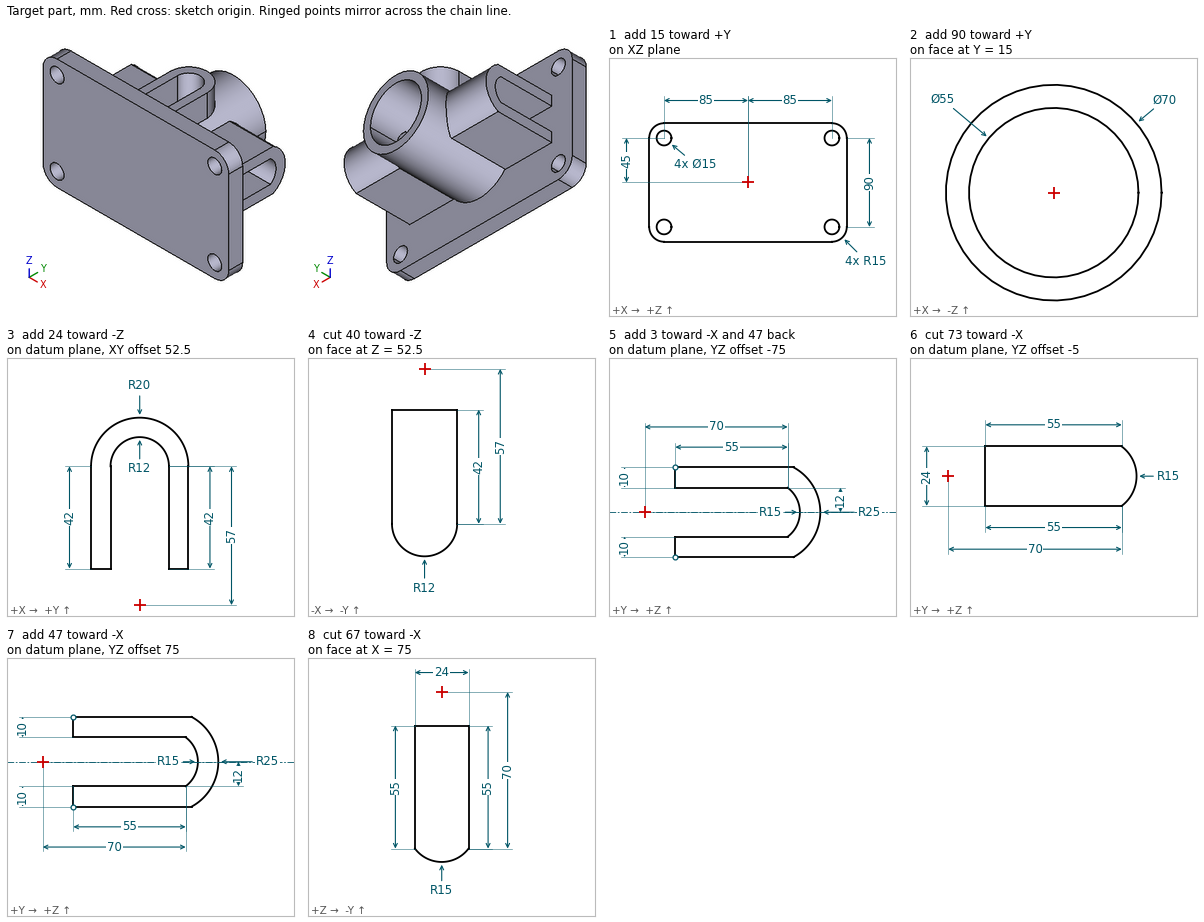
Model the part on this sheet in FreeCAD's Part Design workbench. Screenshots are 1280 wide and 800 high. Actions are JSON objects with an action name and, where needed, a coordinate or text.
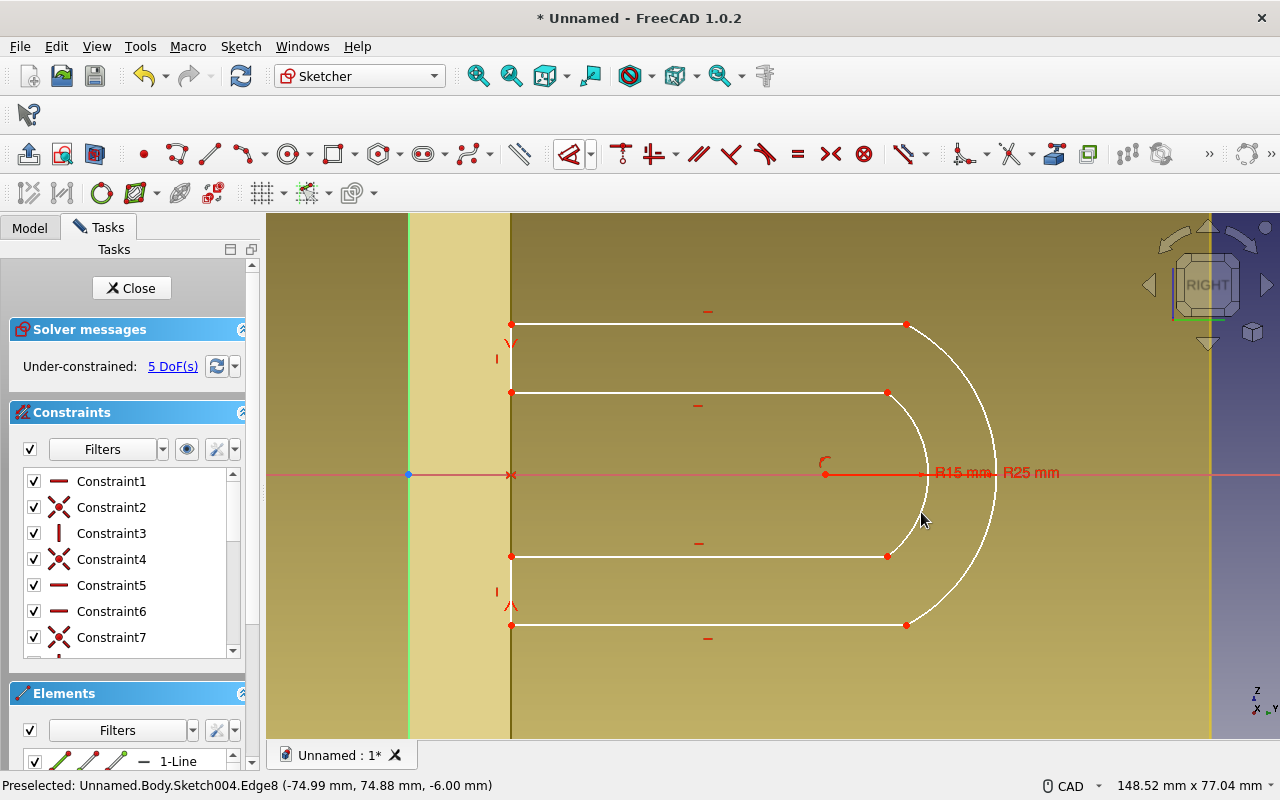
{"action": "left_click", "coordinate": [774, 393]}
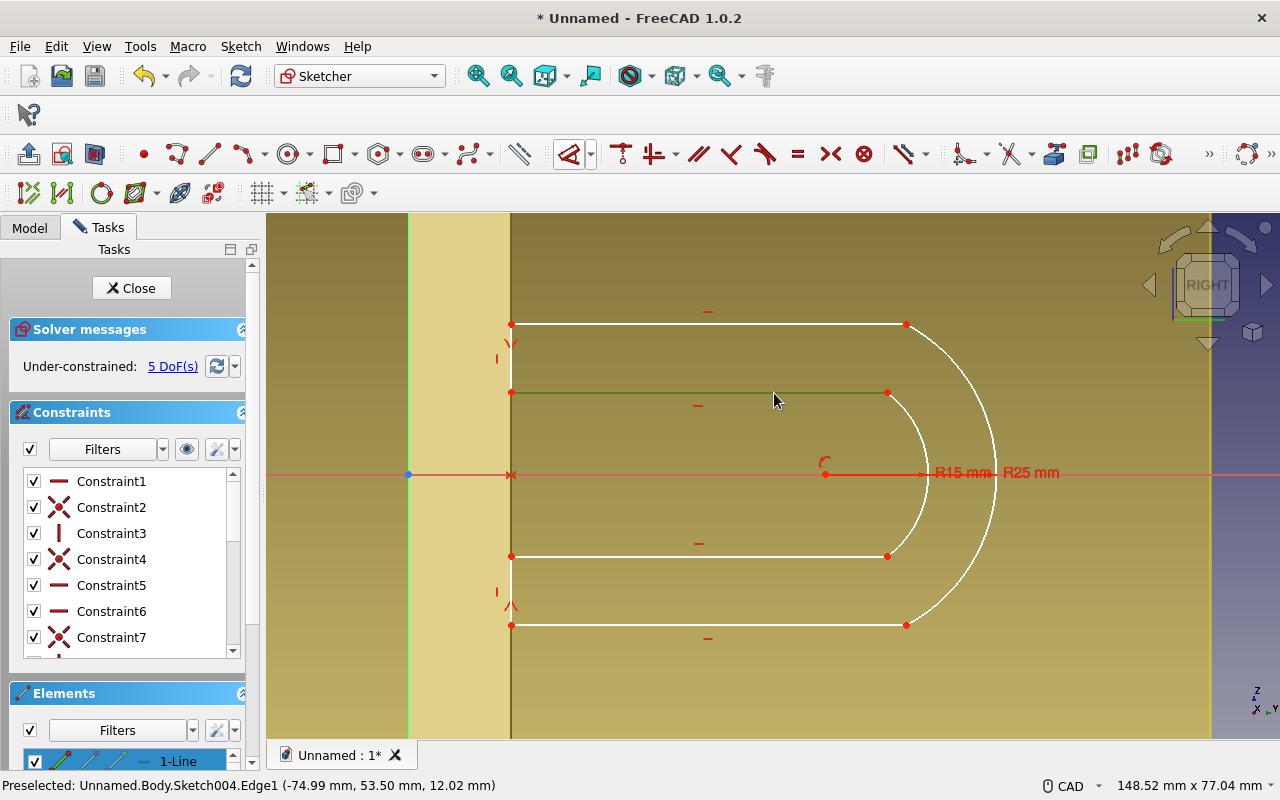
{"action": "key", "text": "l"}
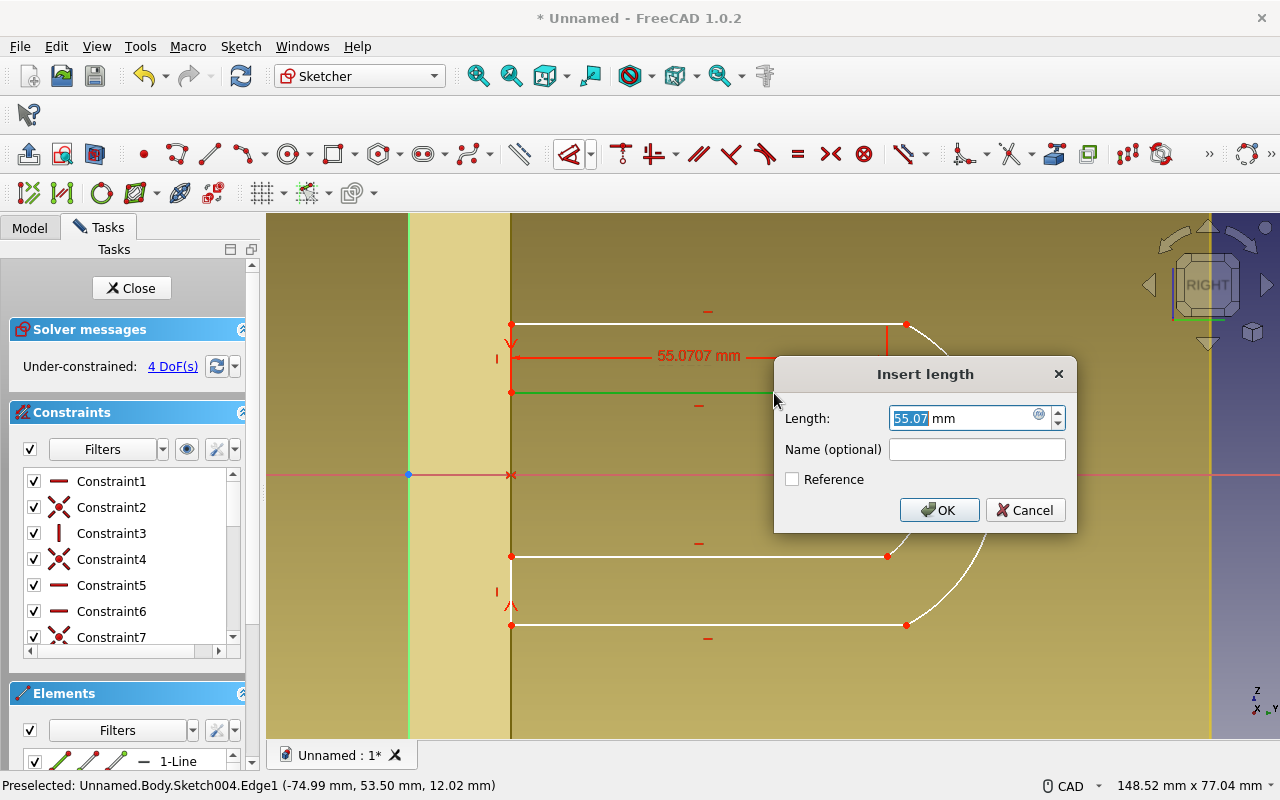
{"action": "type", "text": "55"}
{"action": "key", "text": "Return"}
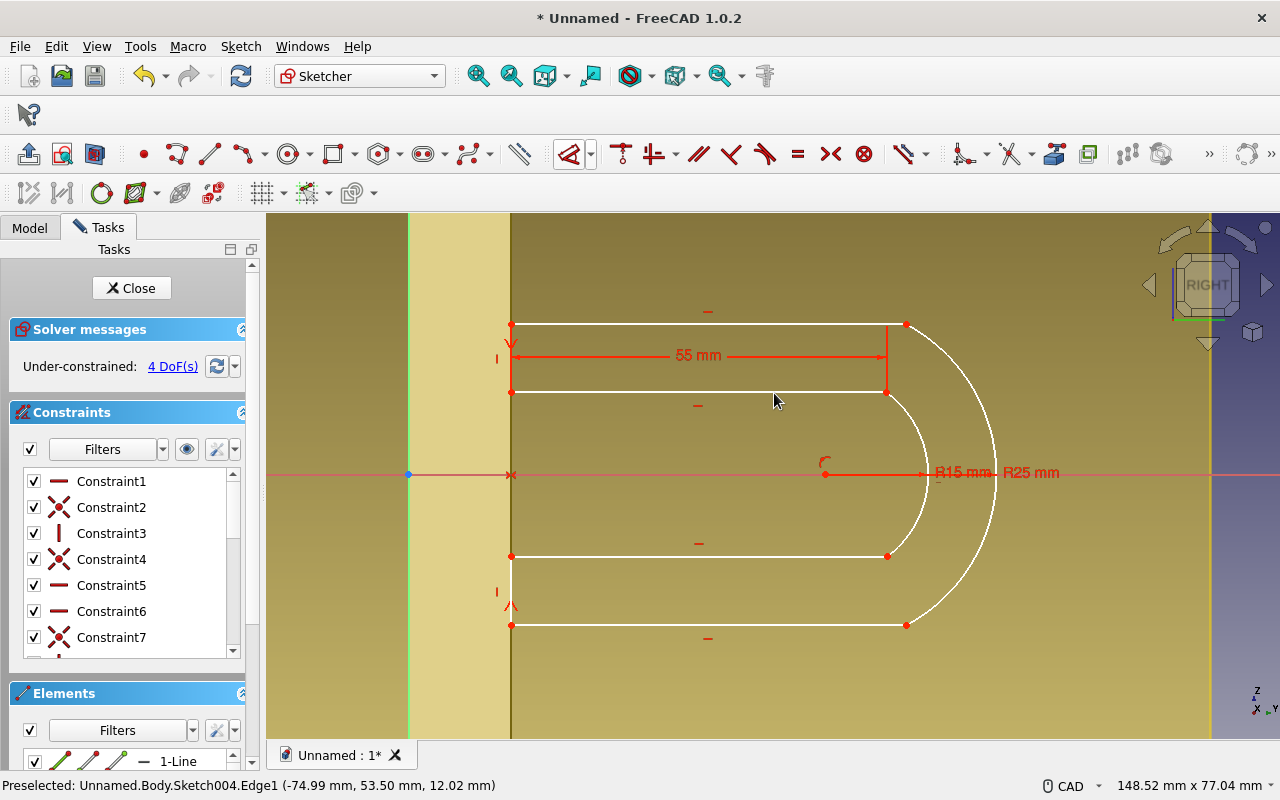
{"action": "left_click", "coordinate": [511, 372]}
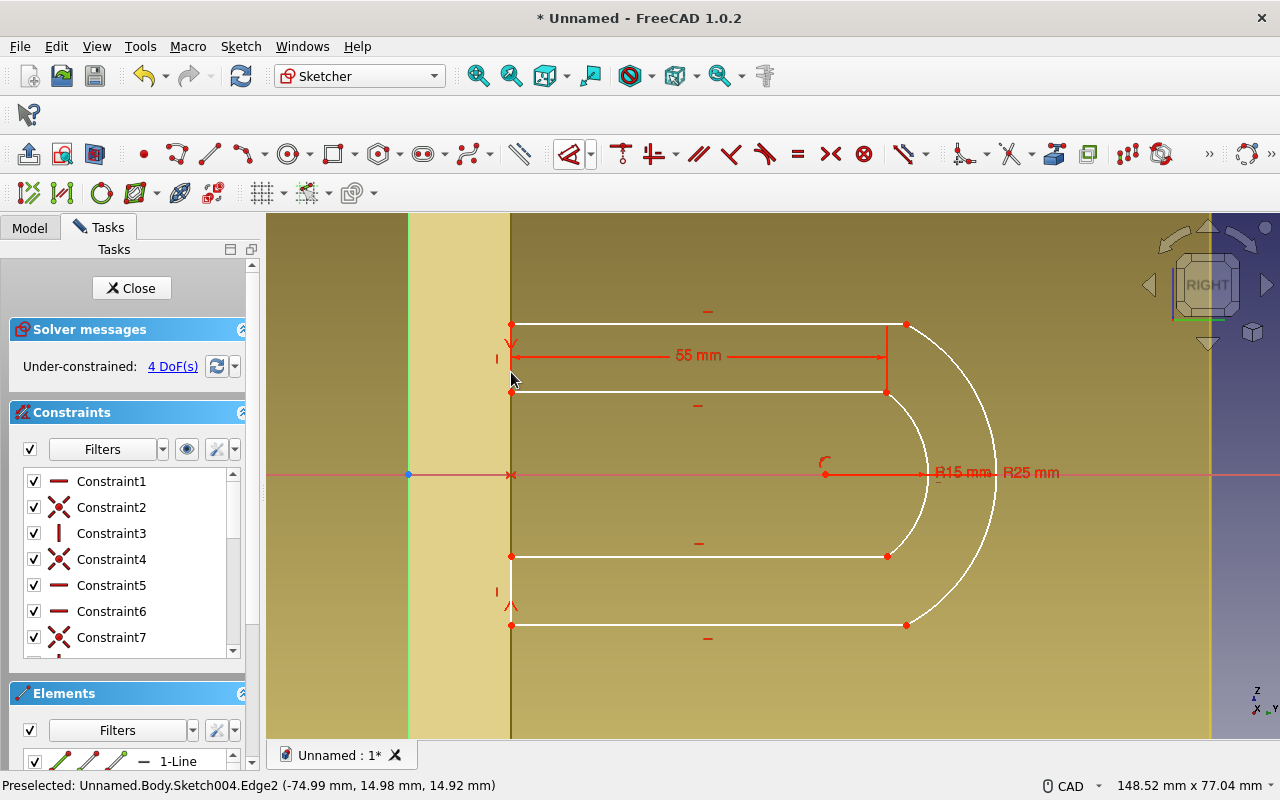
{"action": "key", "text": "i"}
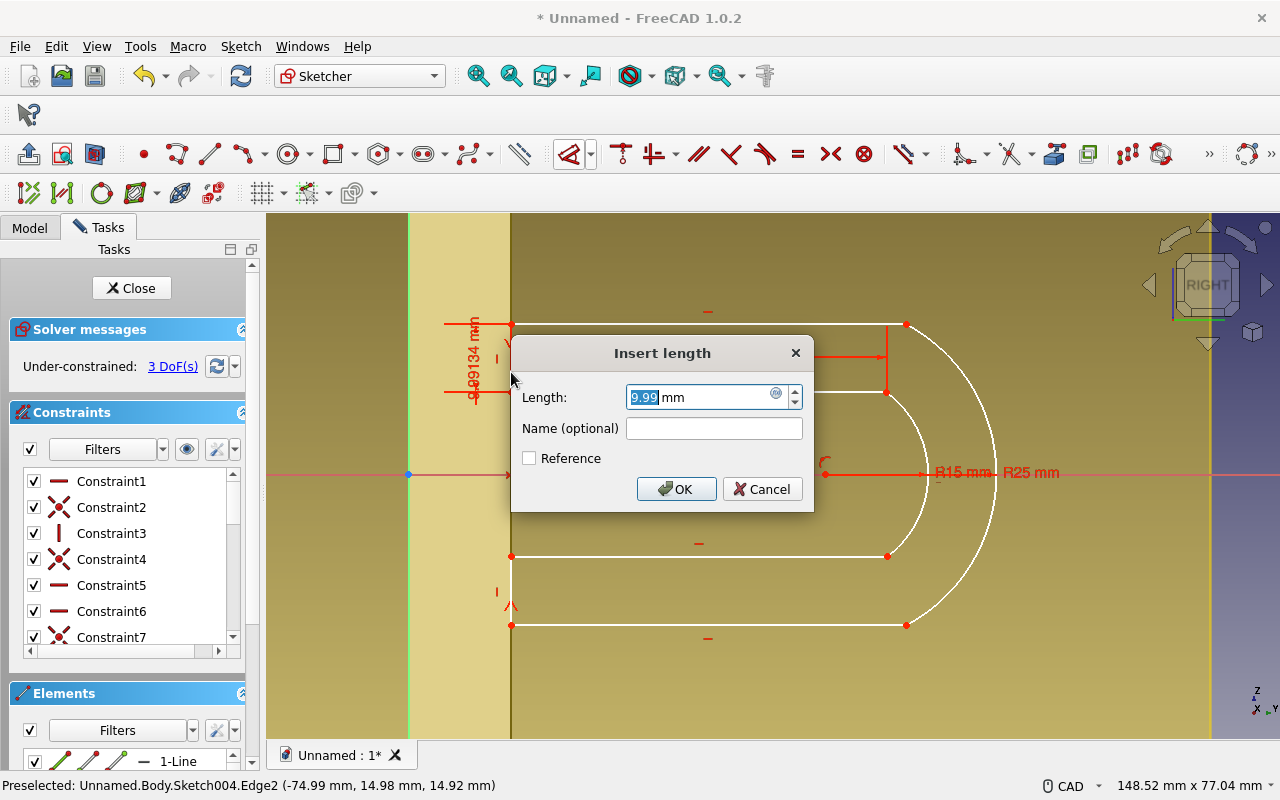
{"action": "type", "text": "10"}
{"action": "key", "text": "Return"}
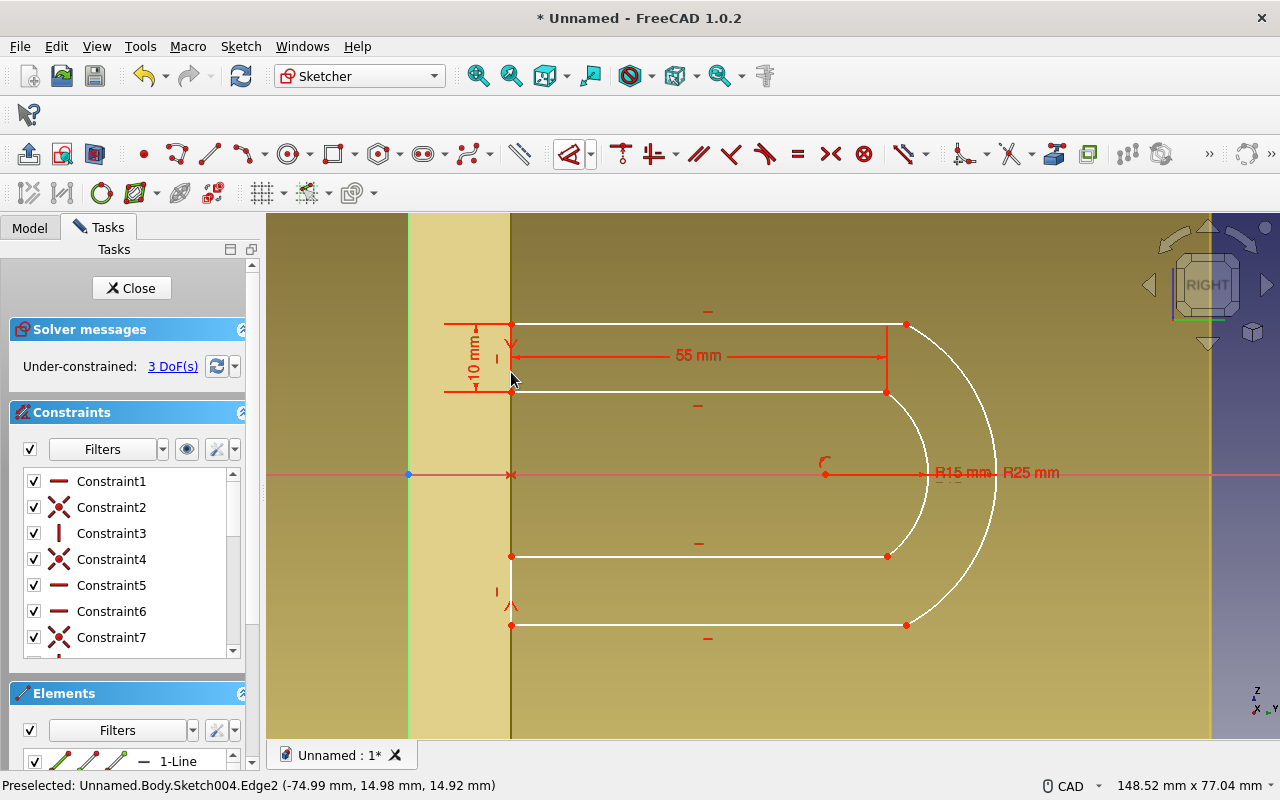
{"action": "left_click", "coordinate": [511, 605]}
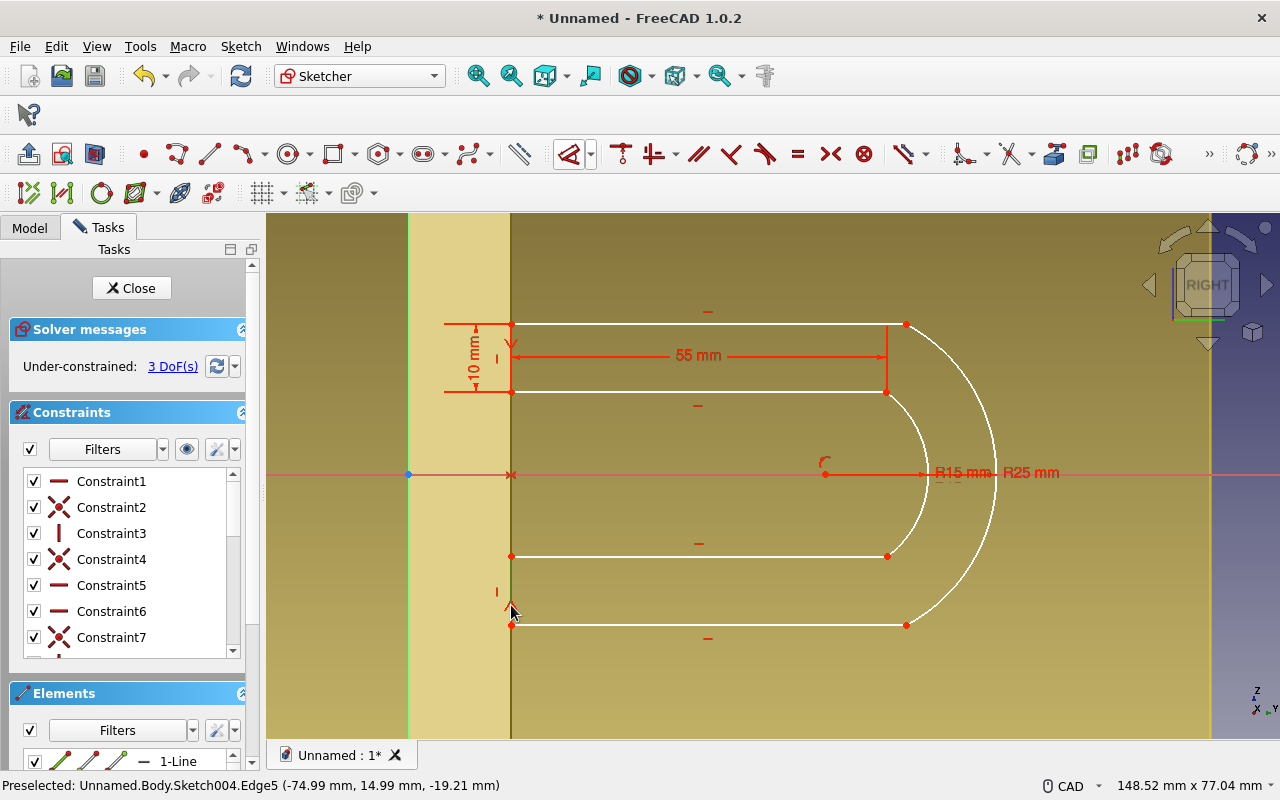
{"action": "key", "text": "i"}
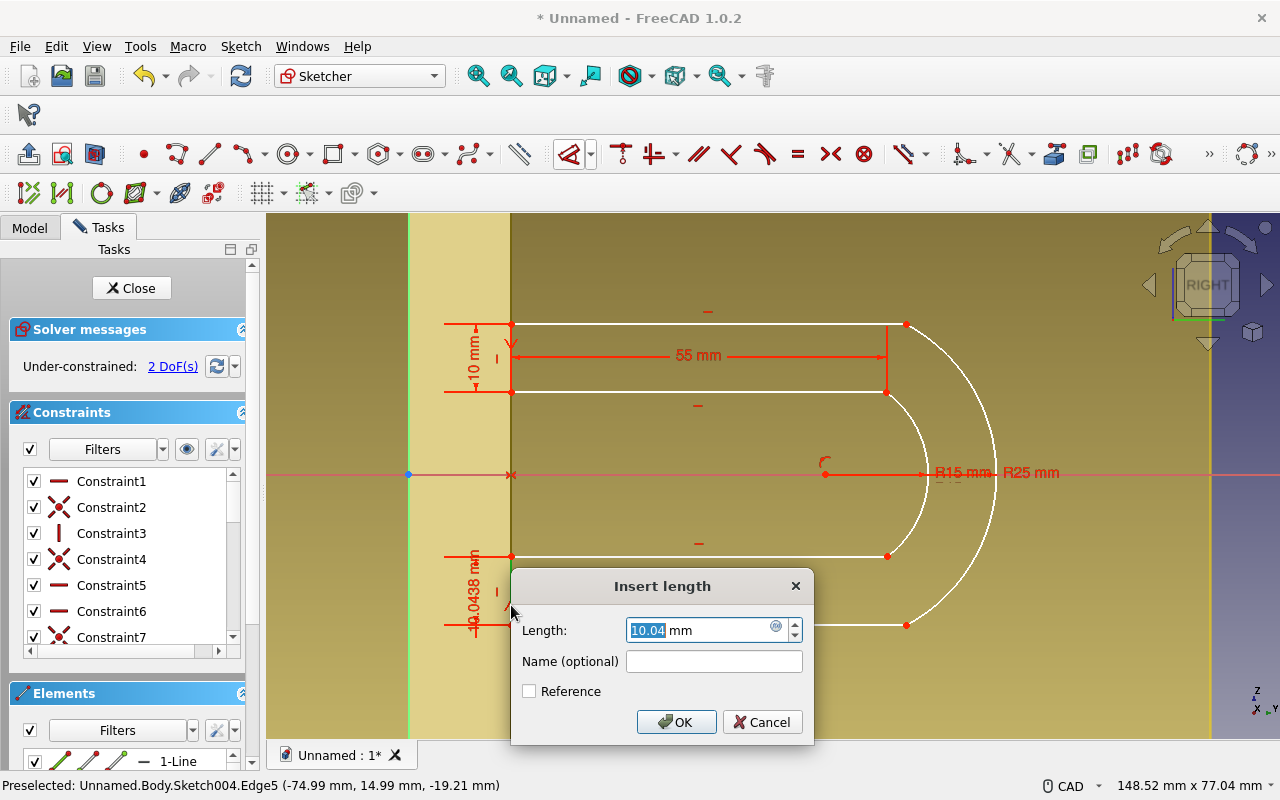
{"action": "type", "text": "10"}
{"action": "key", "text": "Return"}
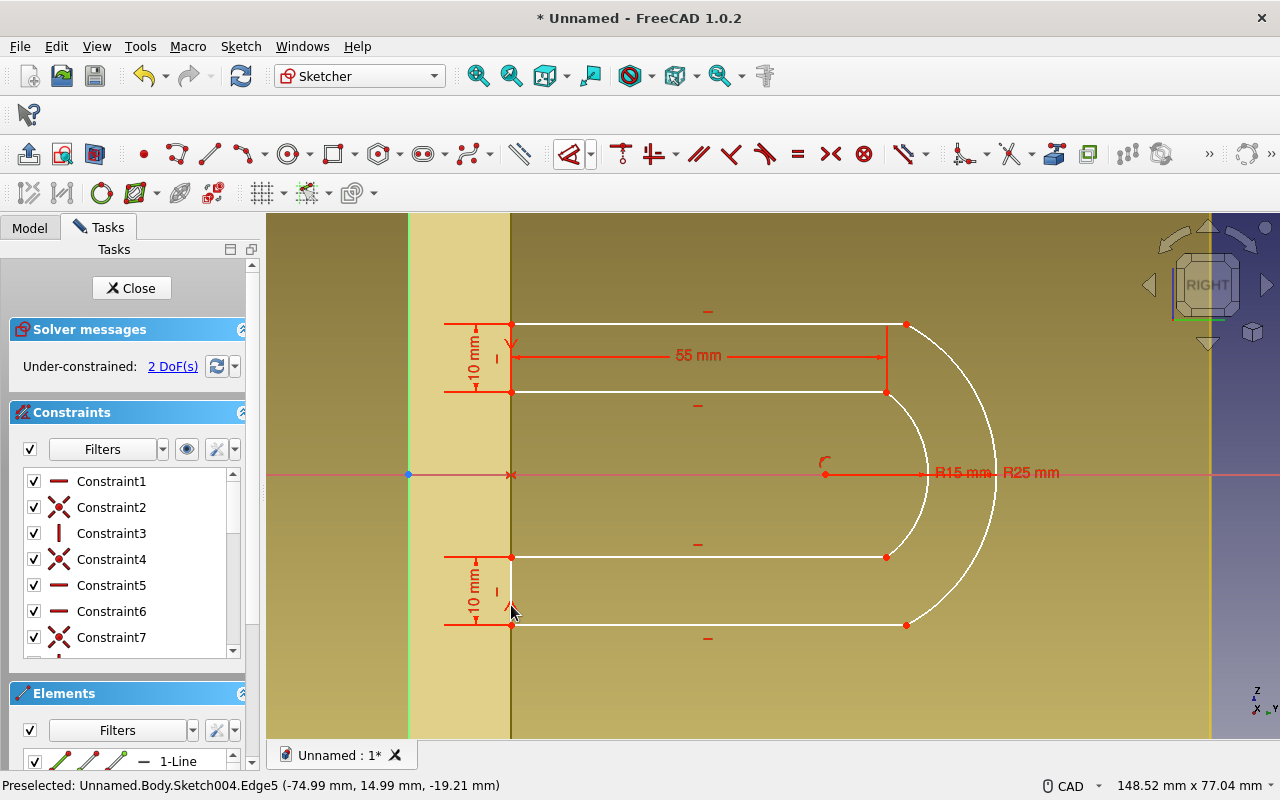
{"action": "left_click", "coordinate": [887, 392]}